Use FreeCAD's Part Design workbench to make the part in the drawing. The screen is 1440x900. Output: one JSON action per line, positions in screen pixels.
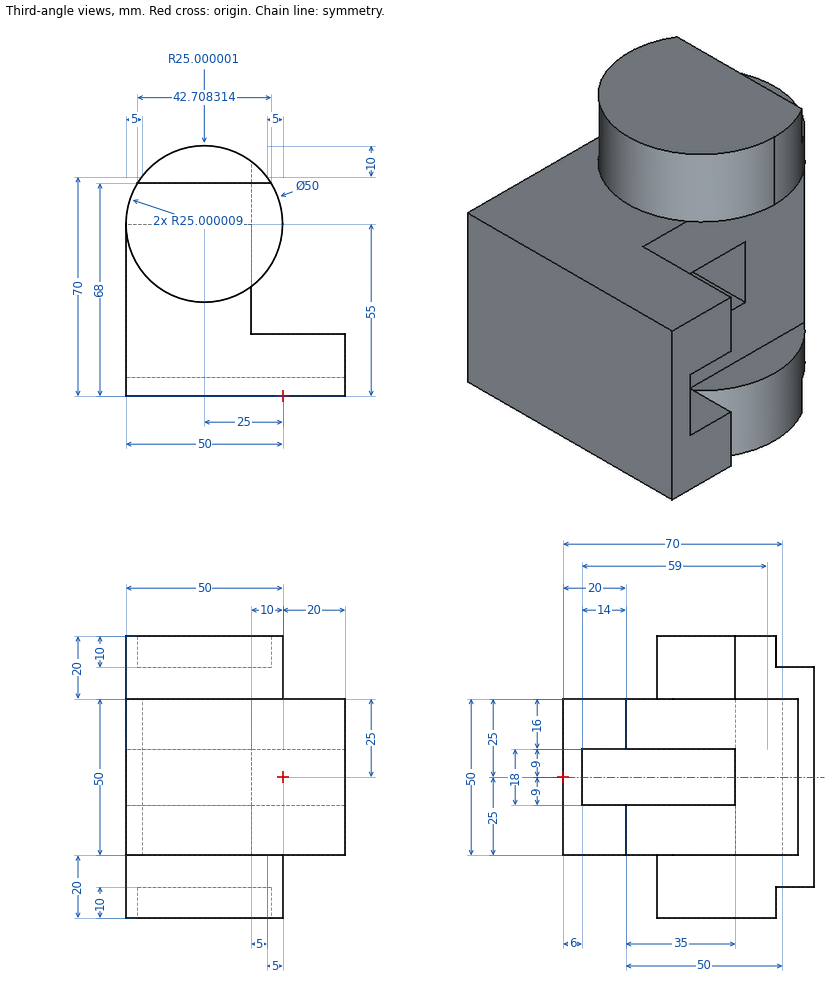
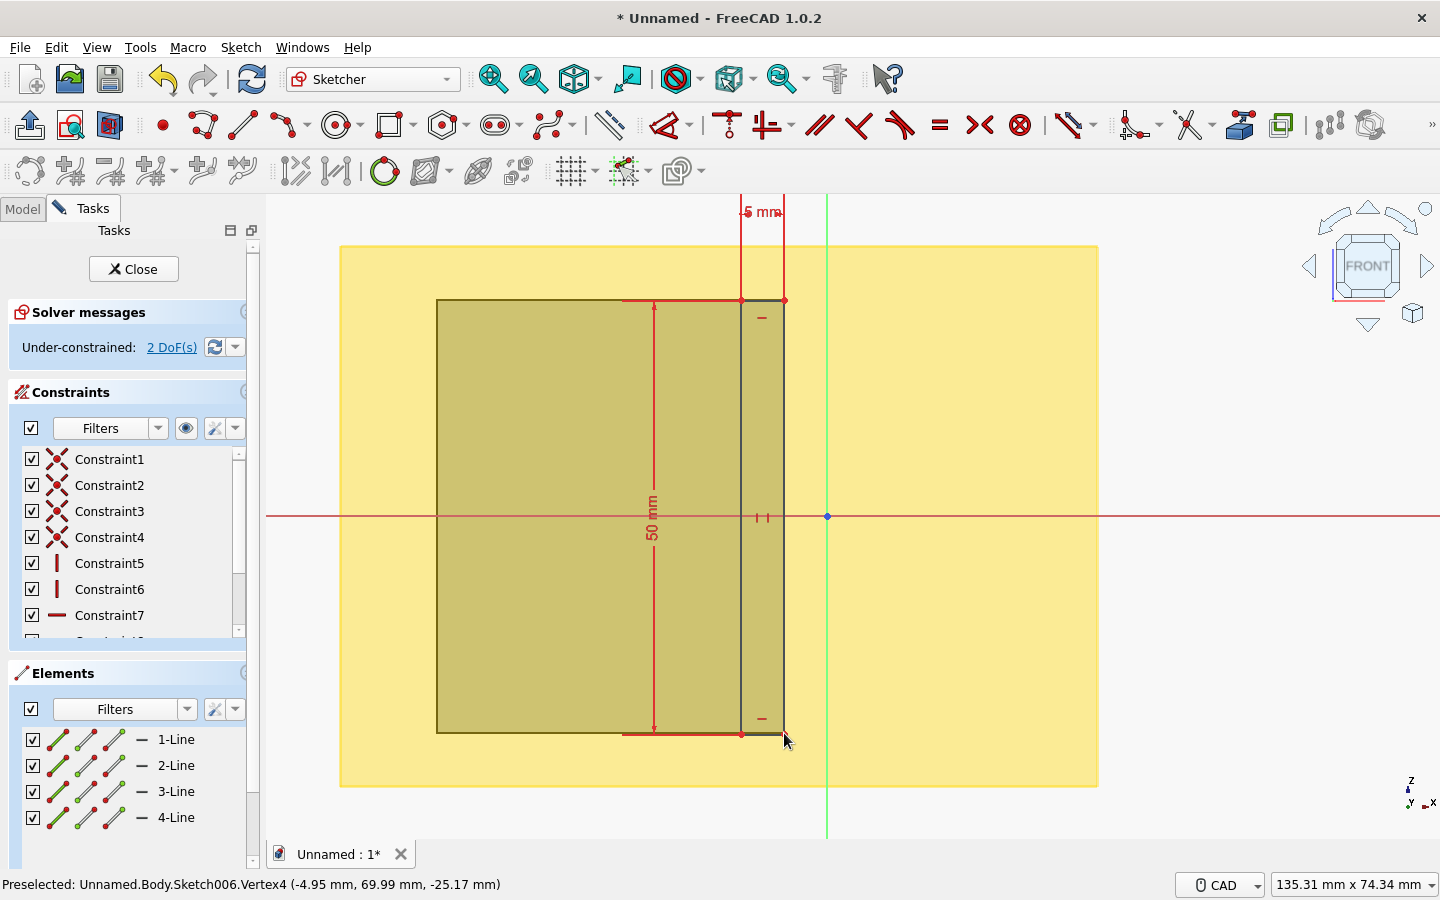
{"action": "left_click", "coordinate": [664, 126]}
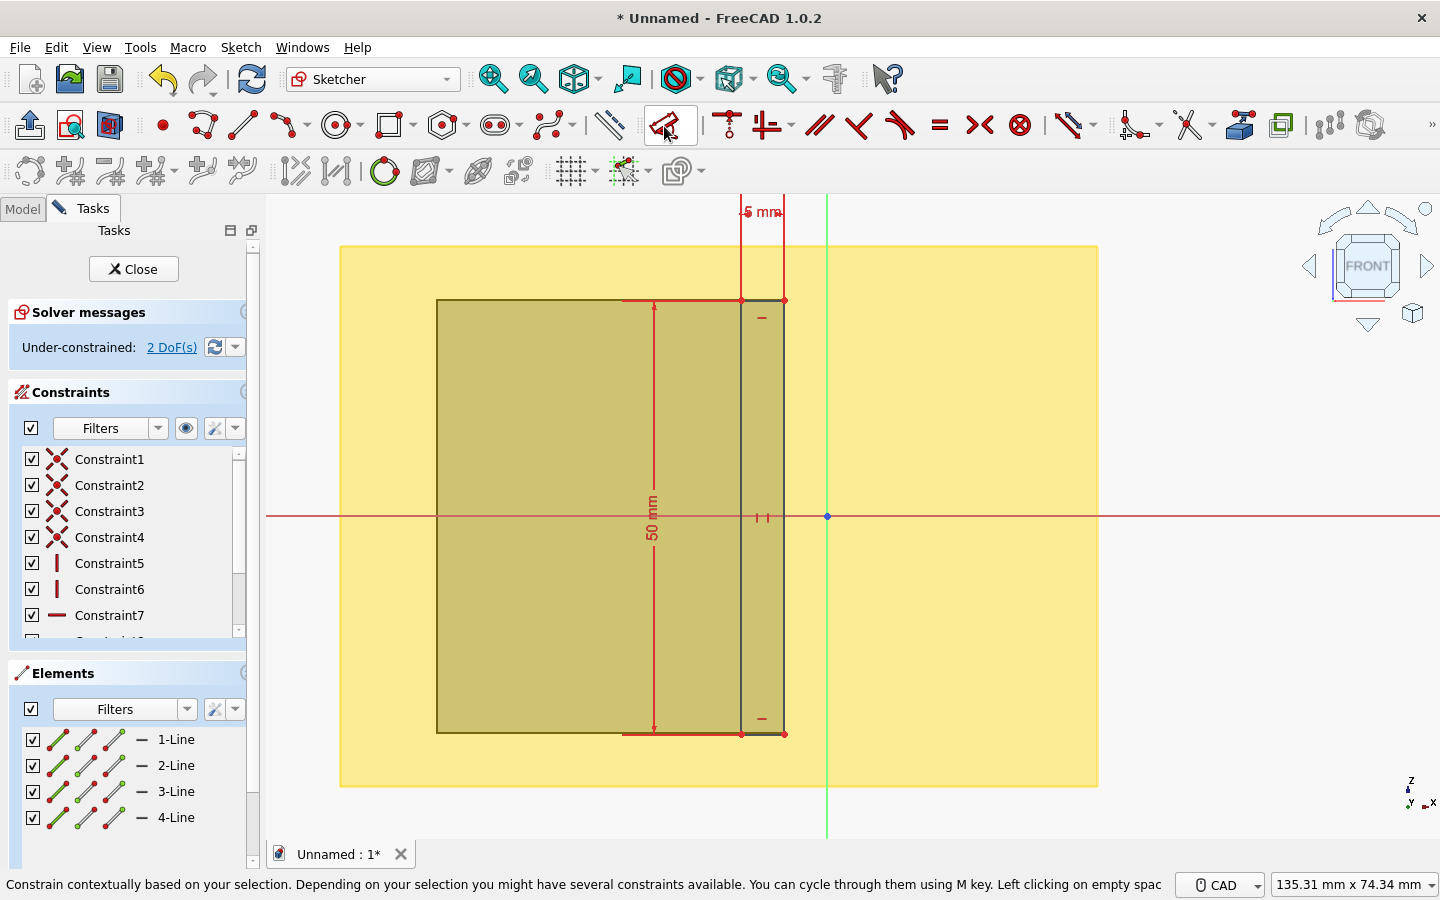
{"action": "left_click", "coordinate": [784, 735]}
{"action": "left_click", "coordinate": [806, 769]}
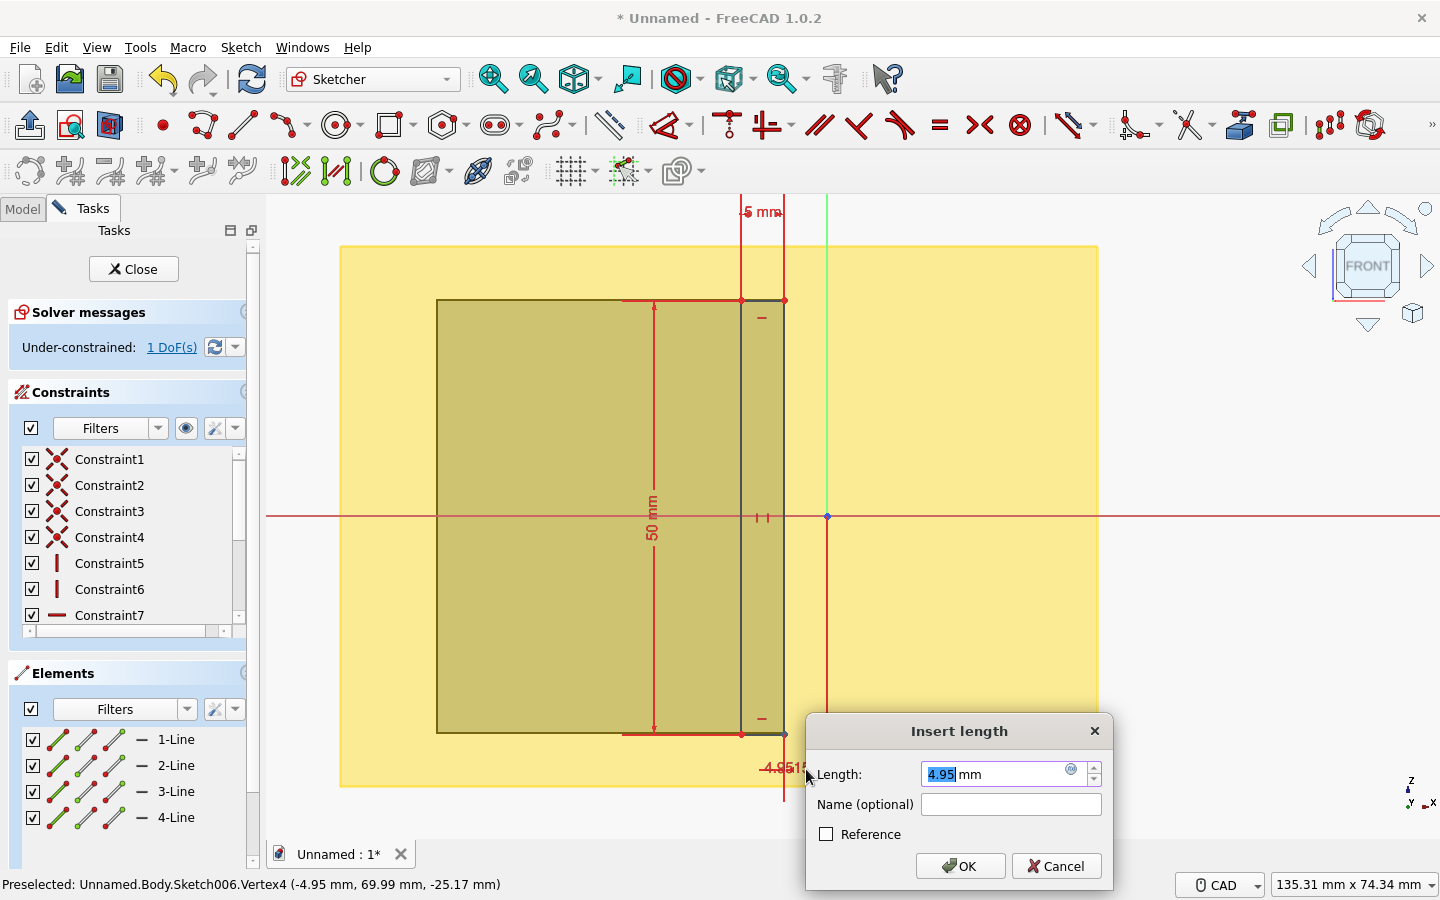
{"action": "type", "text": "5"}
{"action": "key", "text": "Return"}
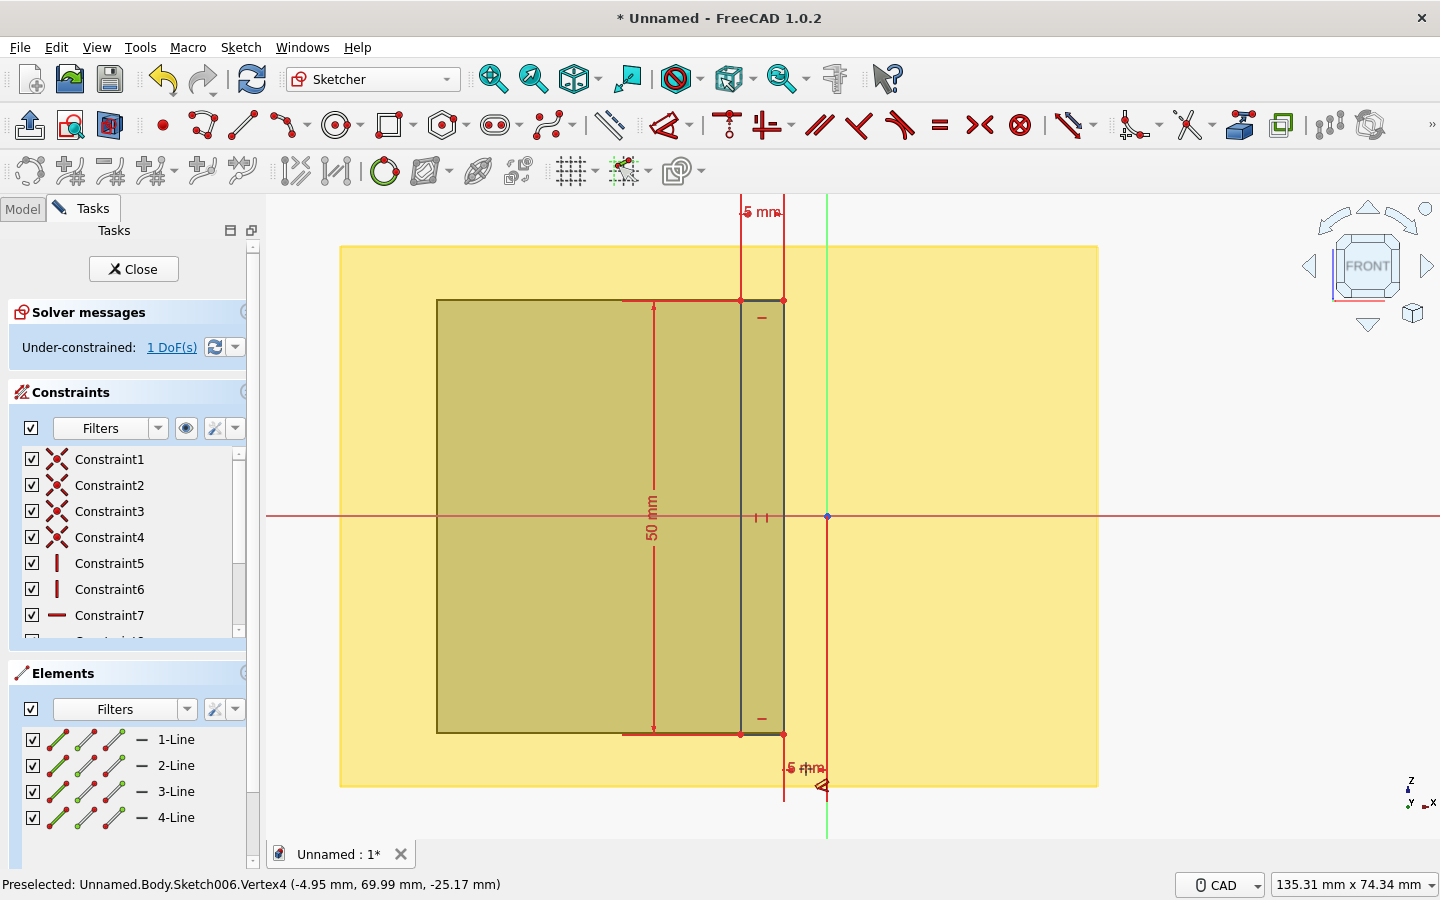
{"action": "left_click", "coordinate": [741, 301]}
{"action": "left_click", "coordinate": [861, 409]}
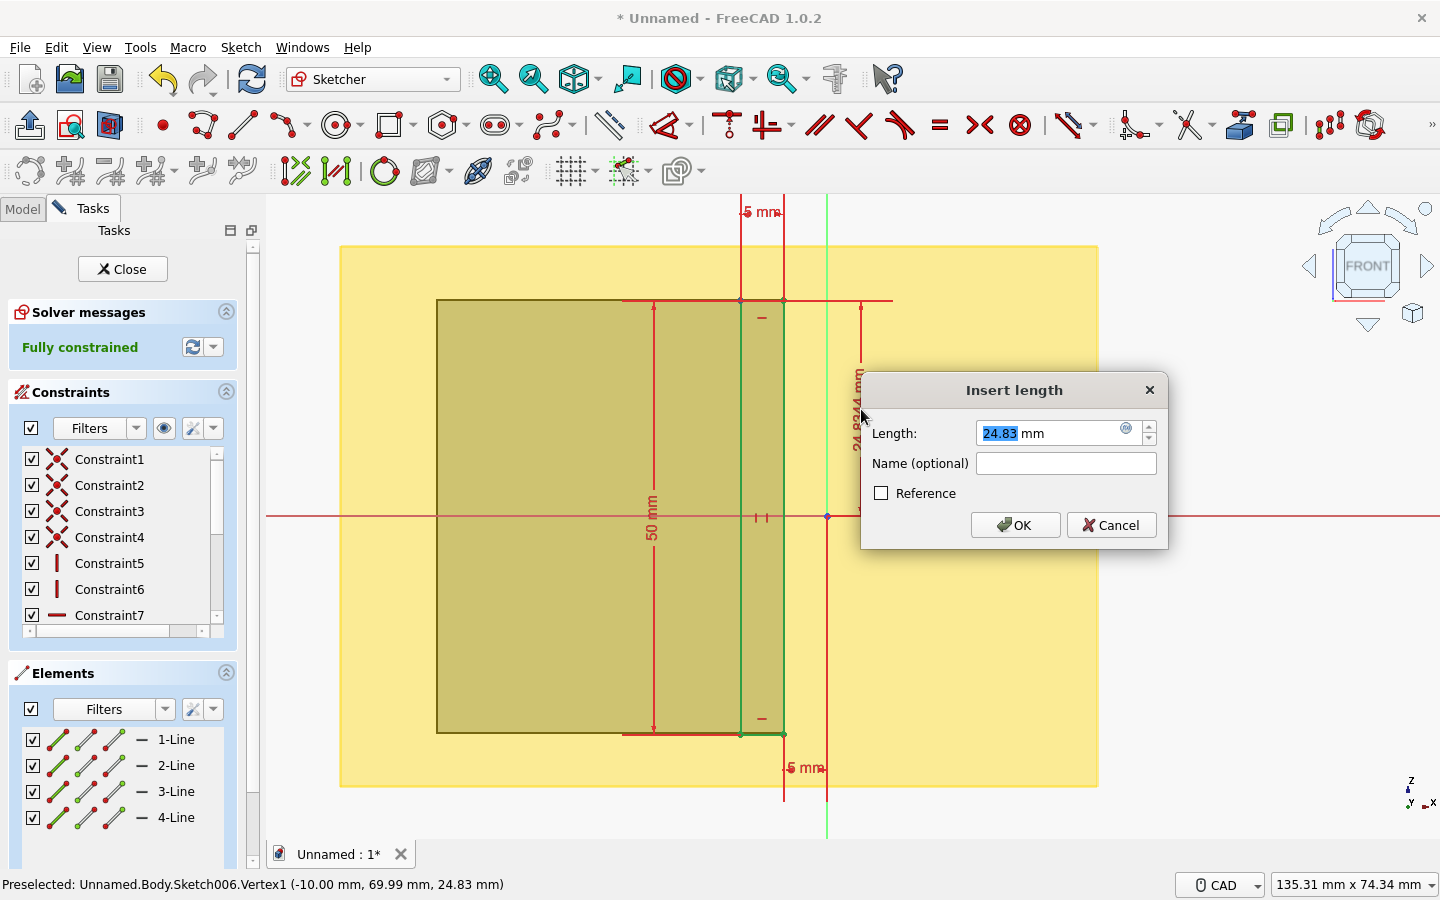
{"action": "type", "text": "25"}
{"action": "key", "text": "Return"}
{"action": "key", "text": "Escape"}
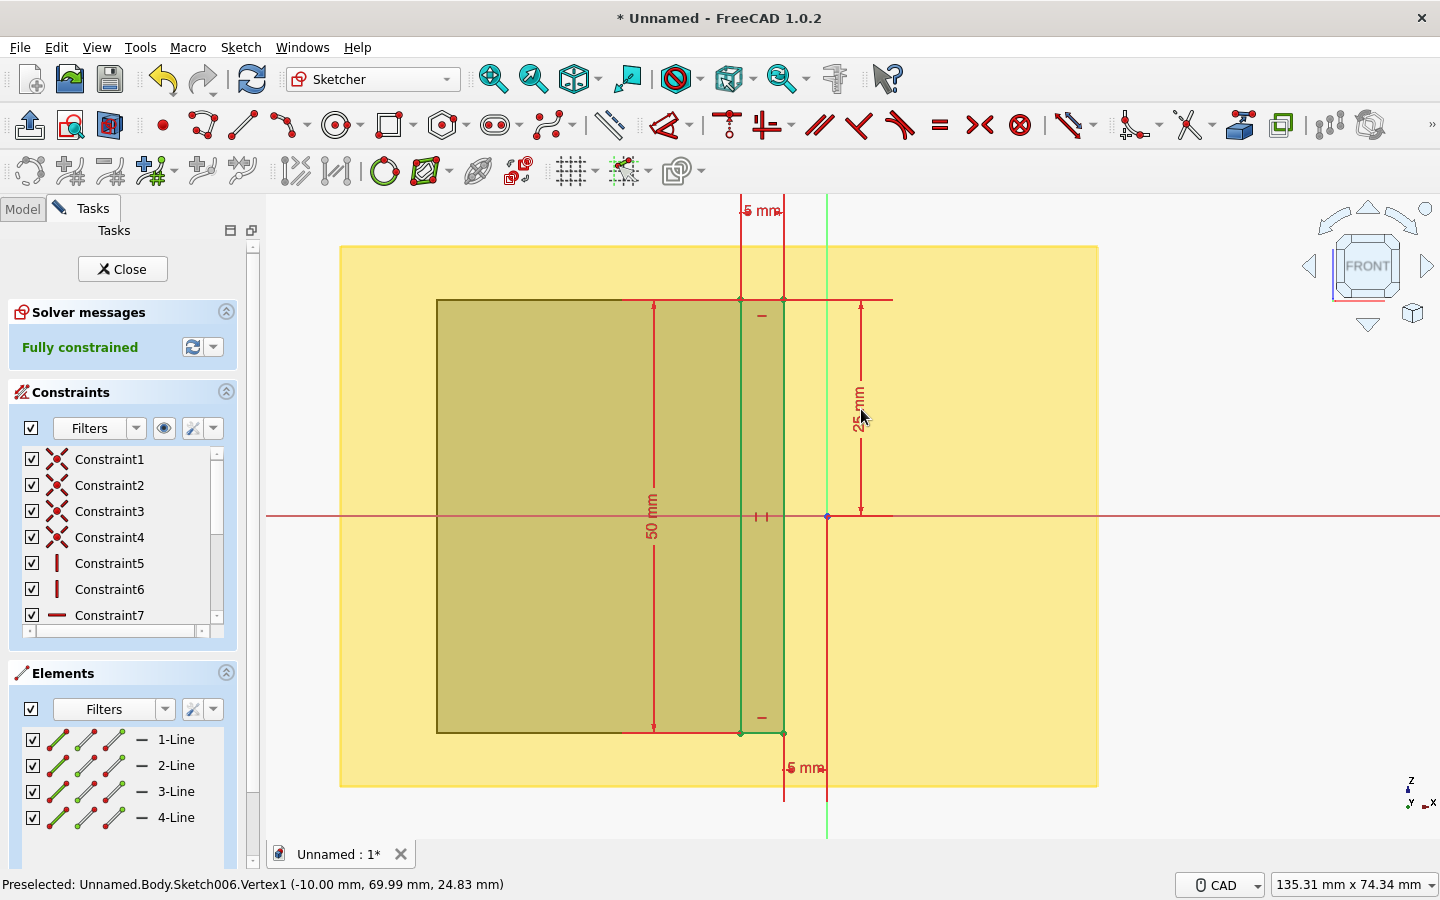
{"action": "left_click", "coordinate": [123, 269]}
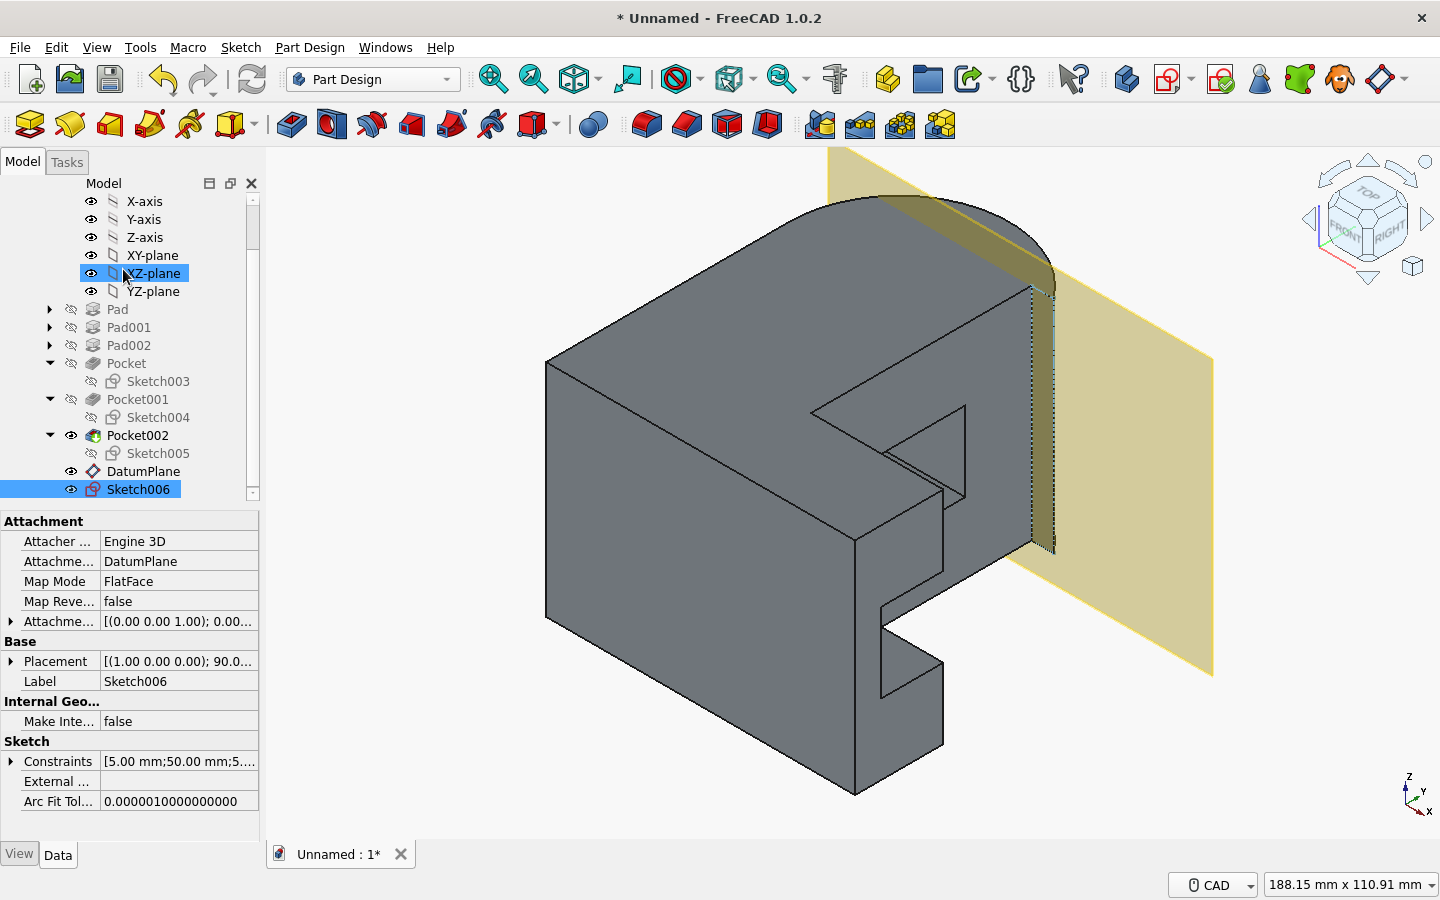
{"action": "left_click", "coordinate": [292, 124]}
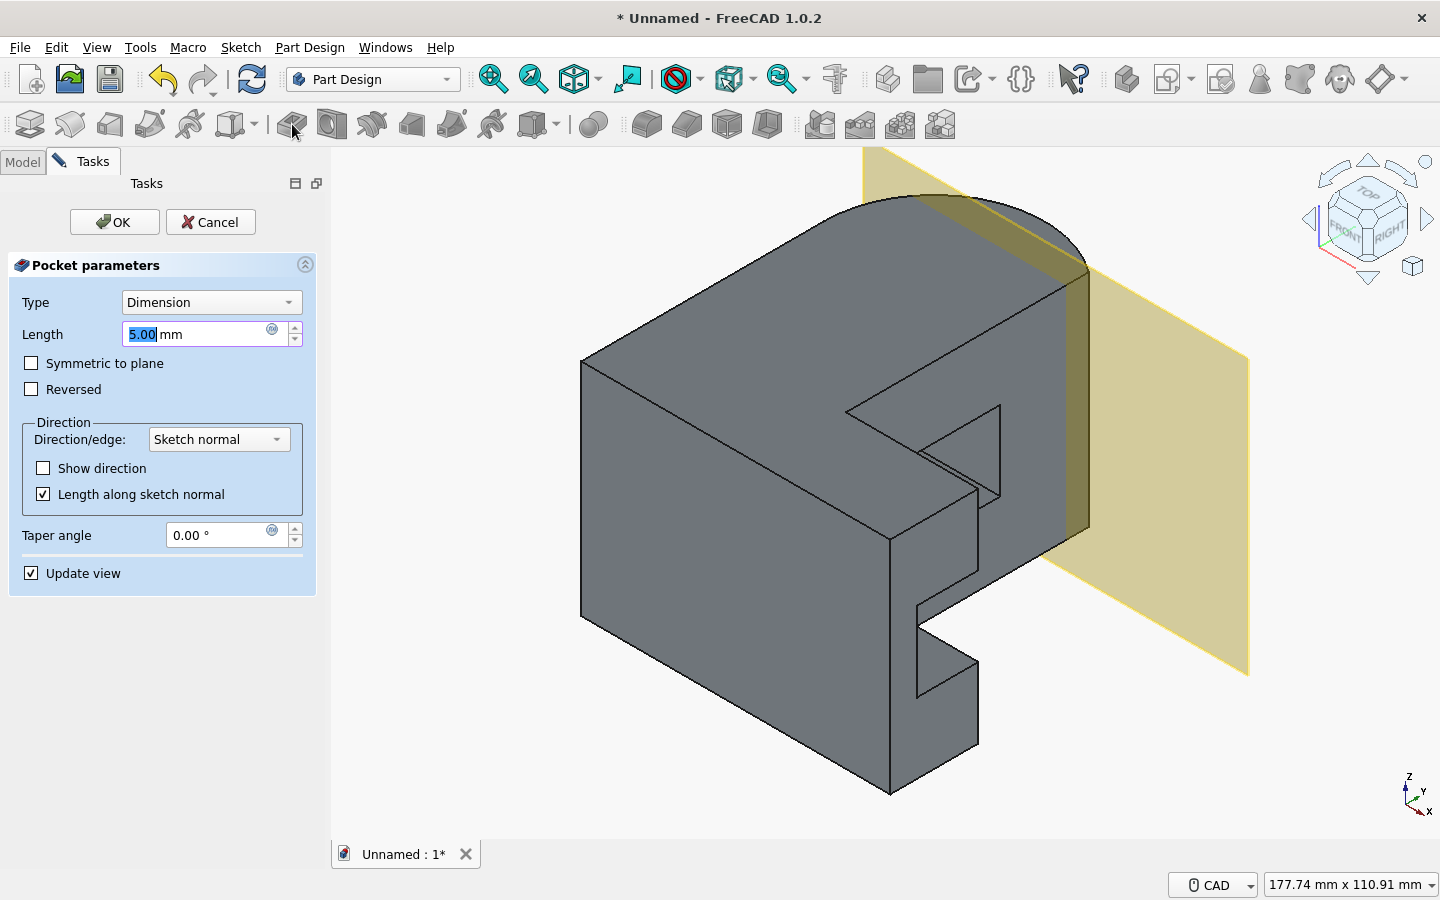
{"action": "type", "text": "10"}
{"action": "key", "text": "Tab"}